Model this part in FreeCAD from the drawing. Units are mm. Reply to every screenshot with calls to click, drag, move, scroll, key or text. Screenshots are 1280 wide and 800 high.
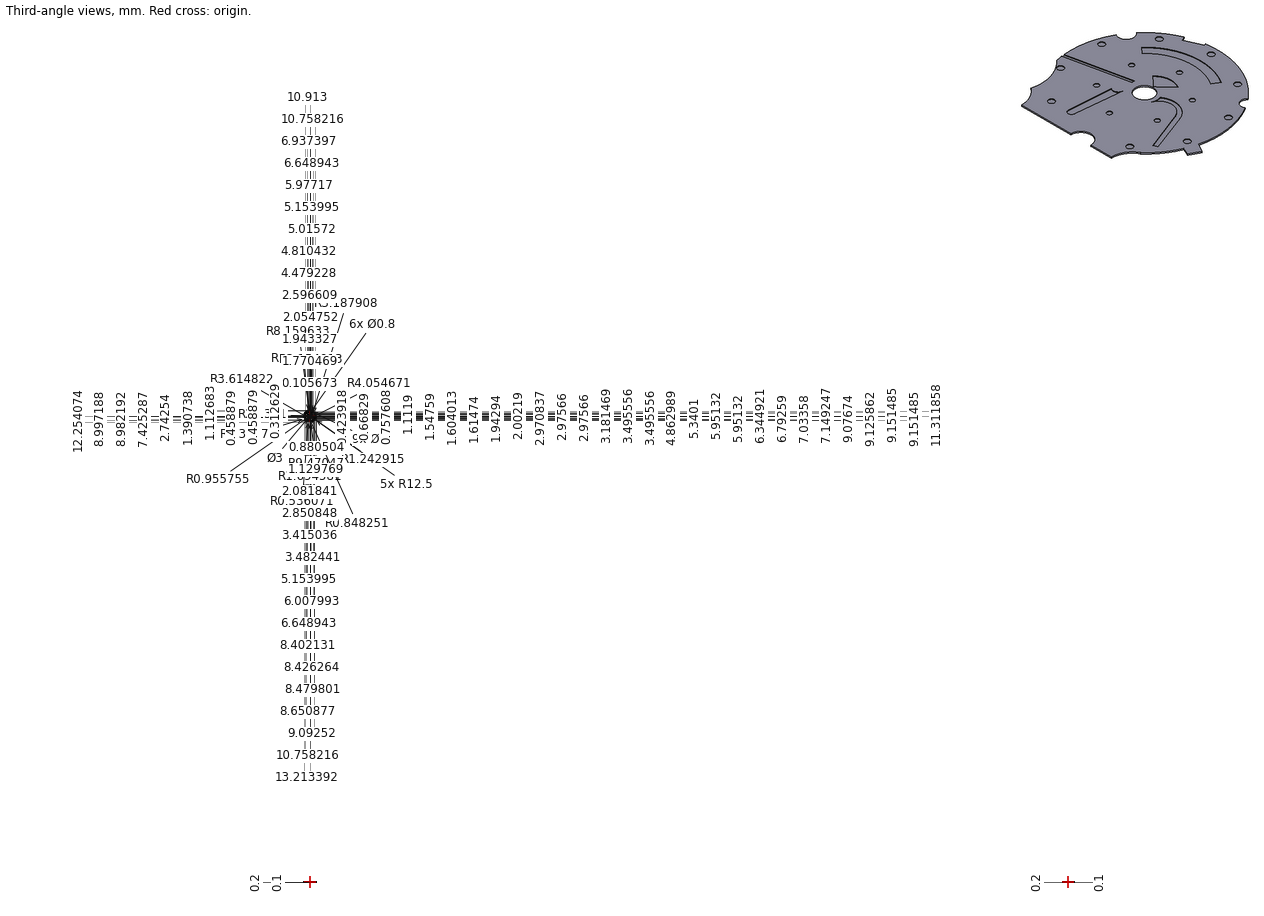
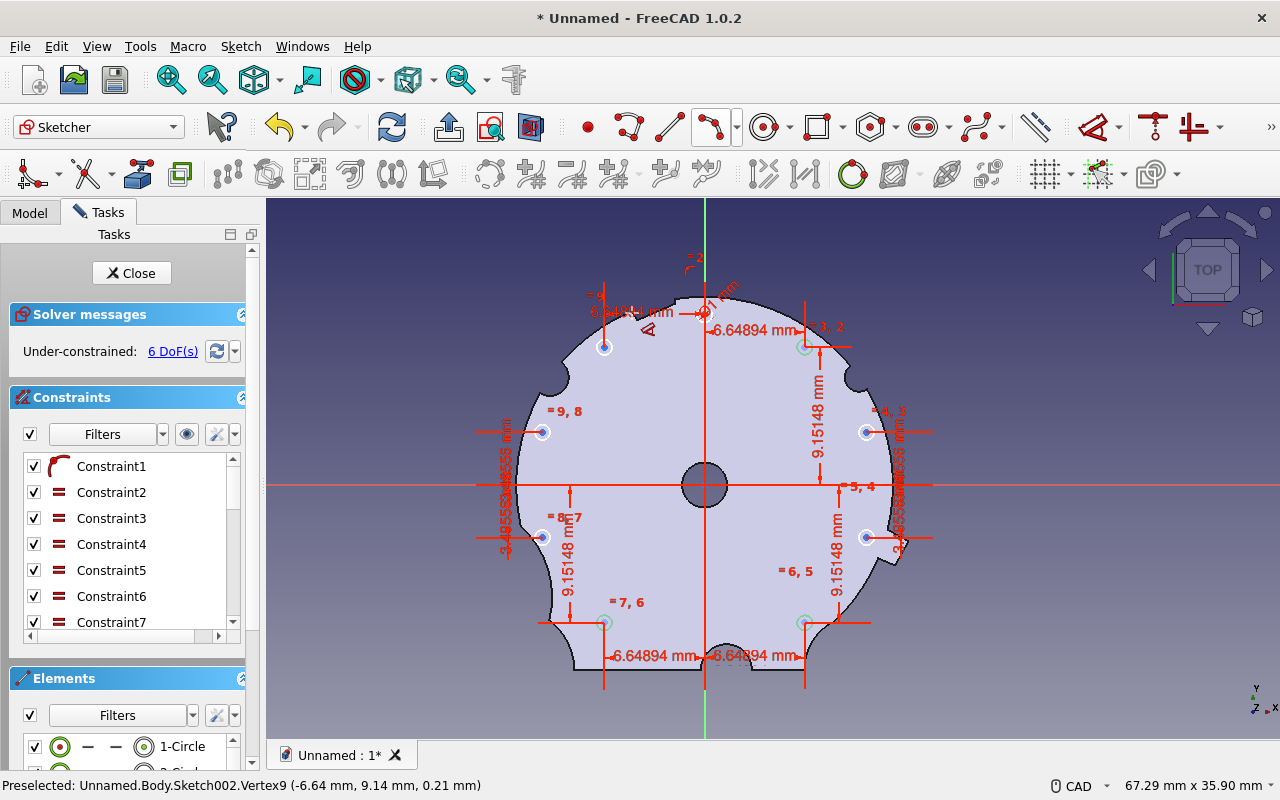
click(604, 347)
click(570, 416)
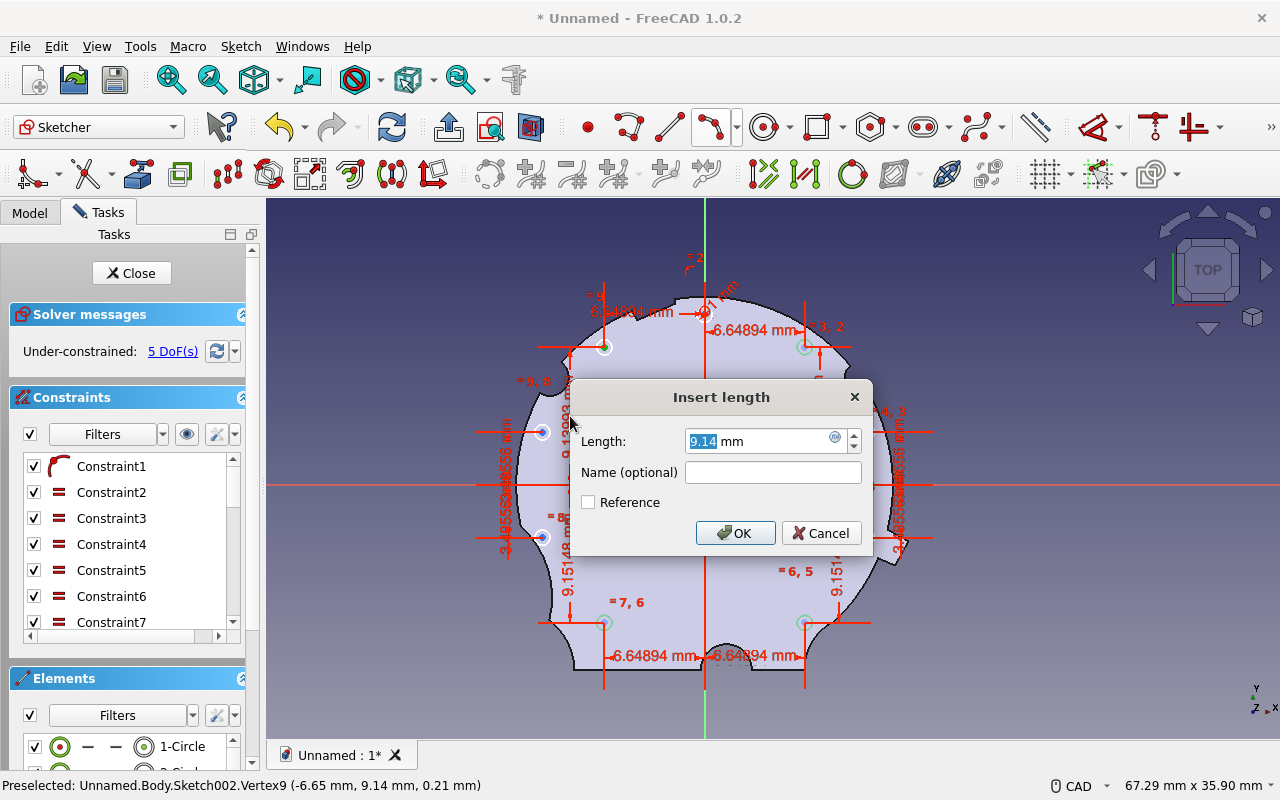
text(9.151485)
key(Return)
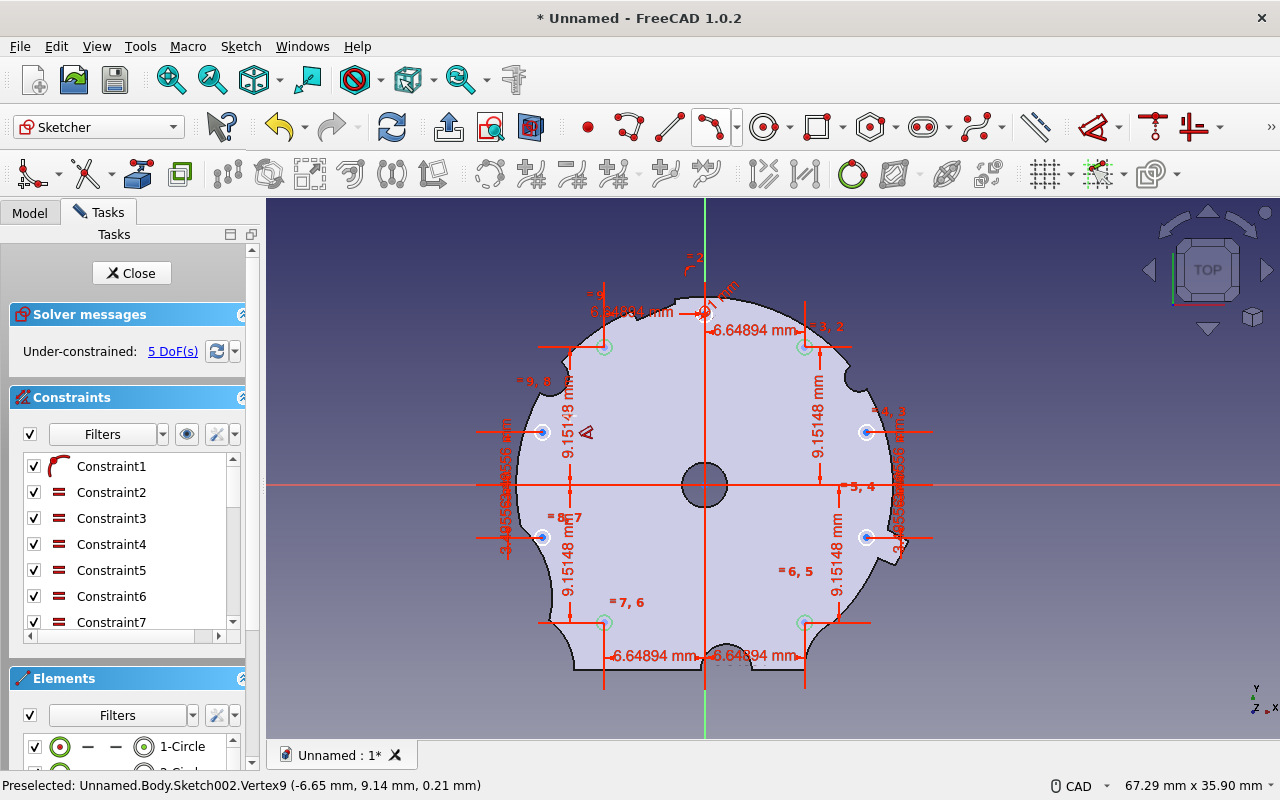
click(705, 315)
click(739, 400)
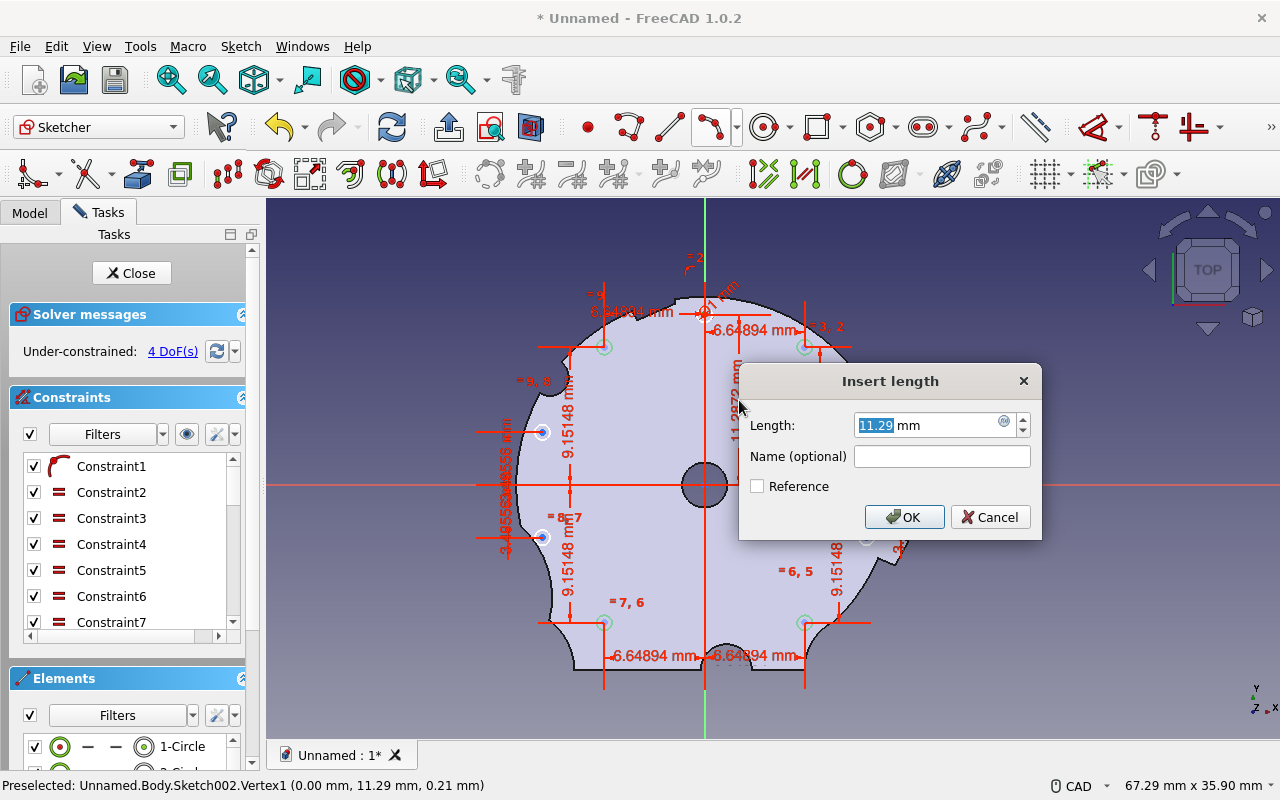
text(11.311858)
key(Return)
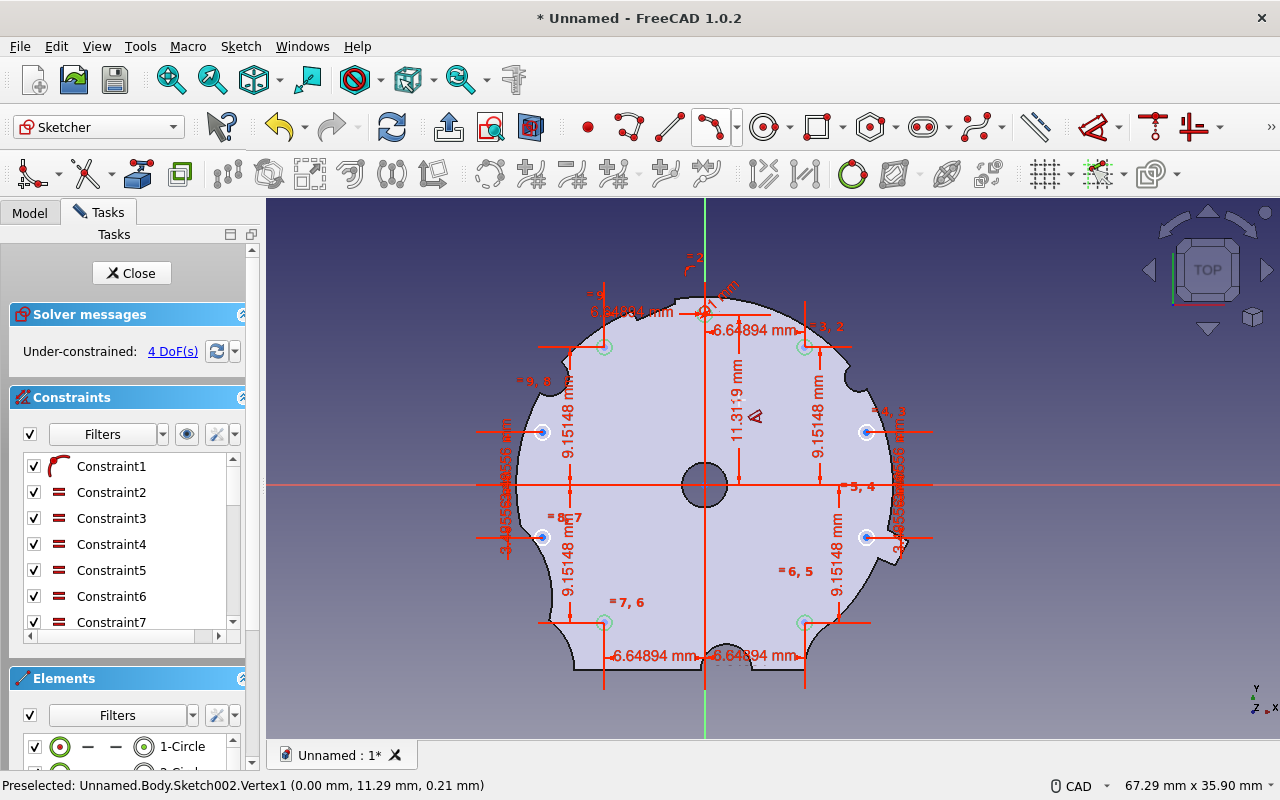
click(867, 432)
click(786, 519)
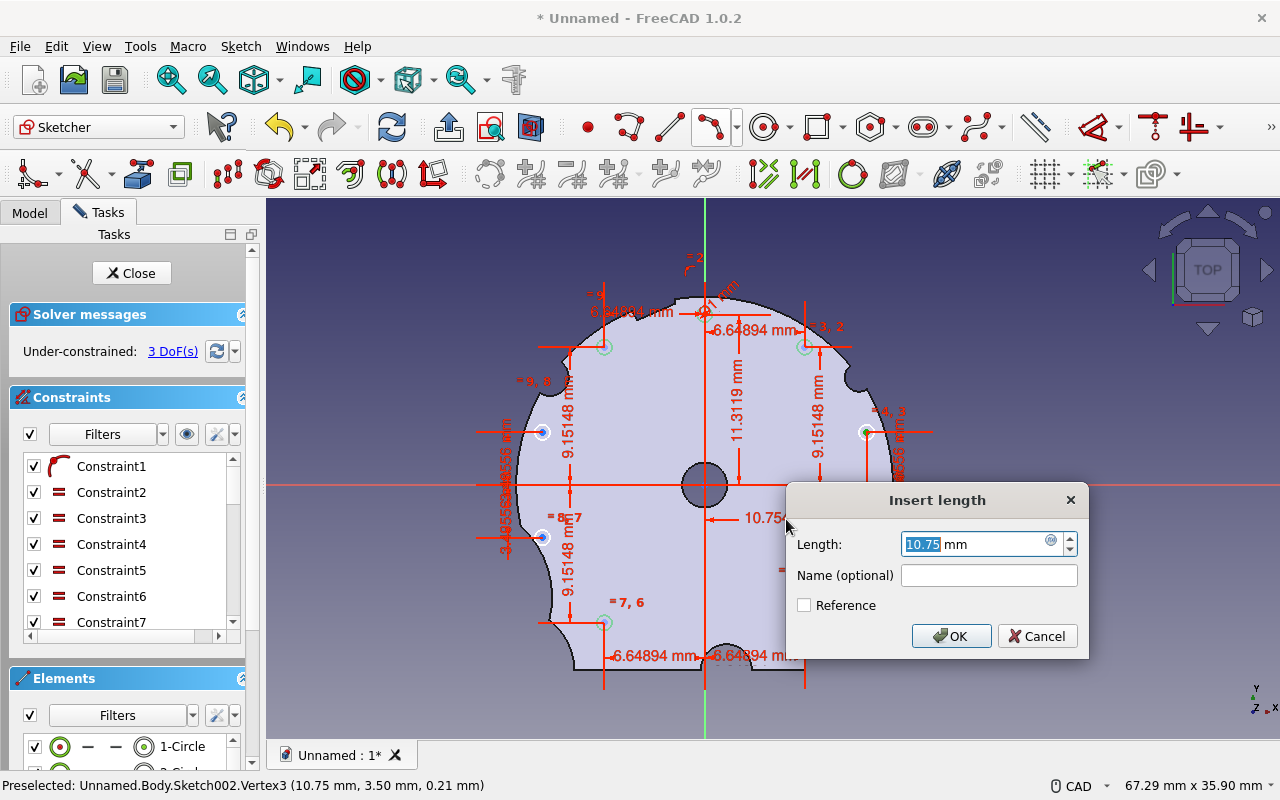
text(10.758216)
key(Return)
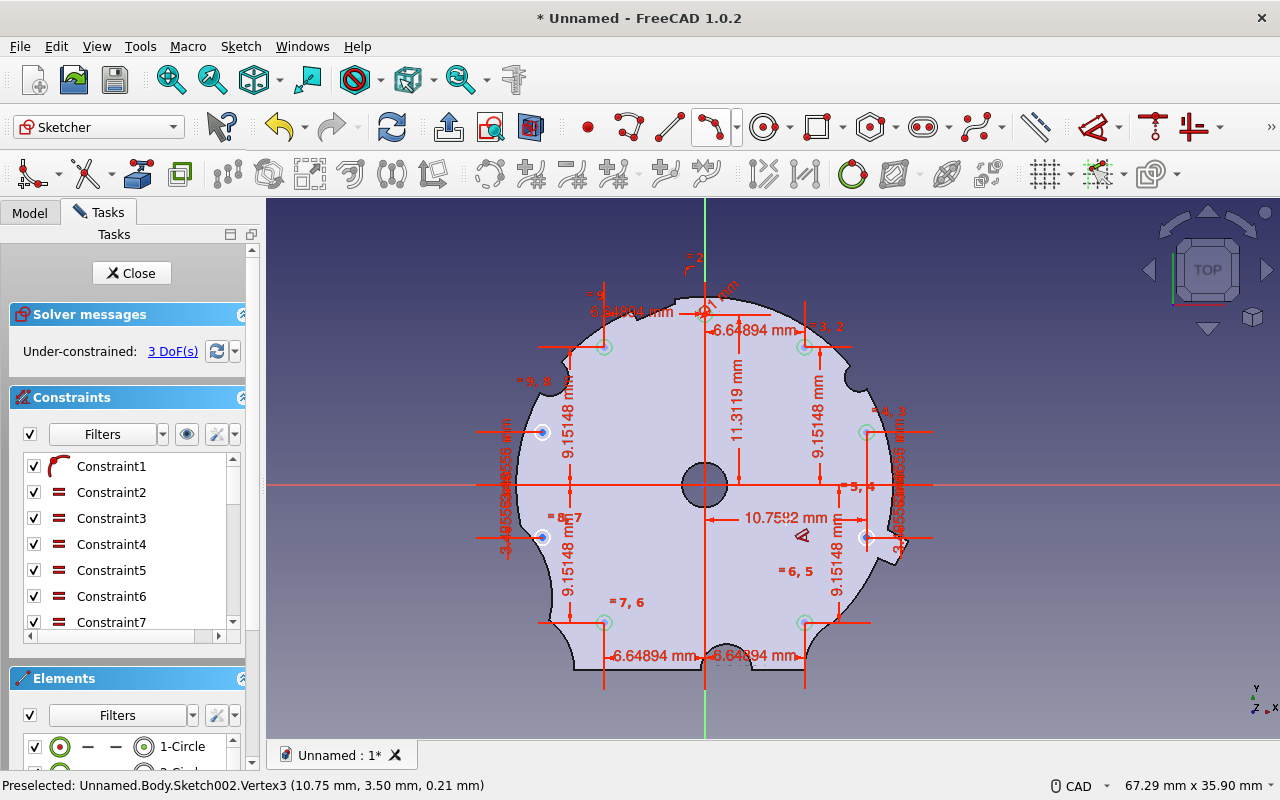
click(867, 538)
click(748, 572)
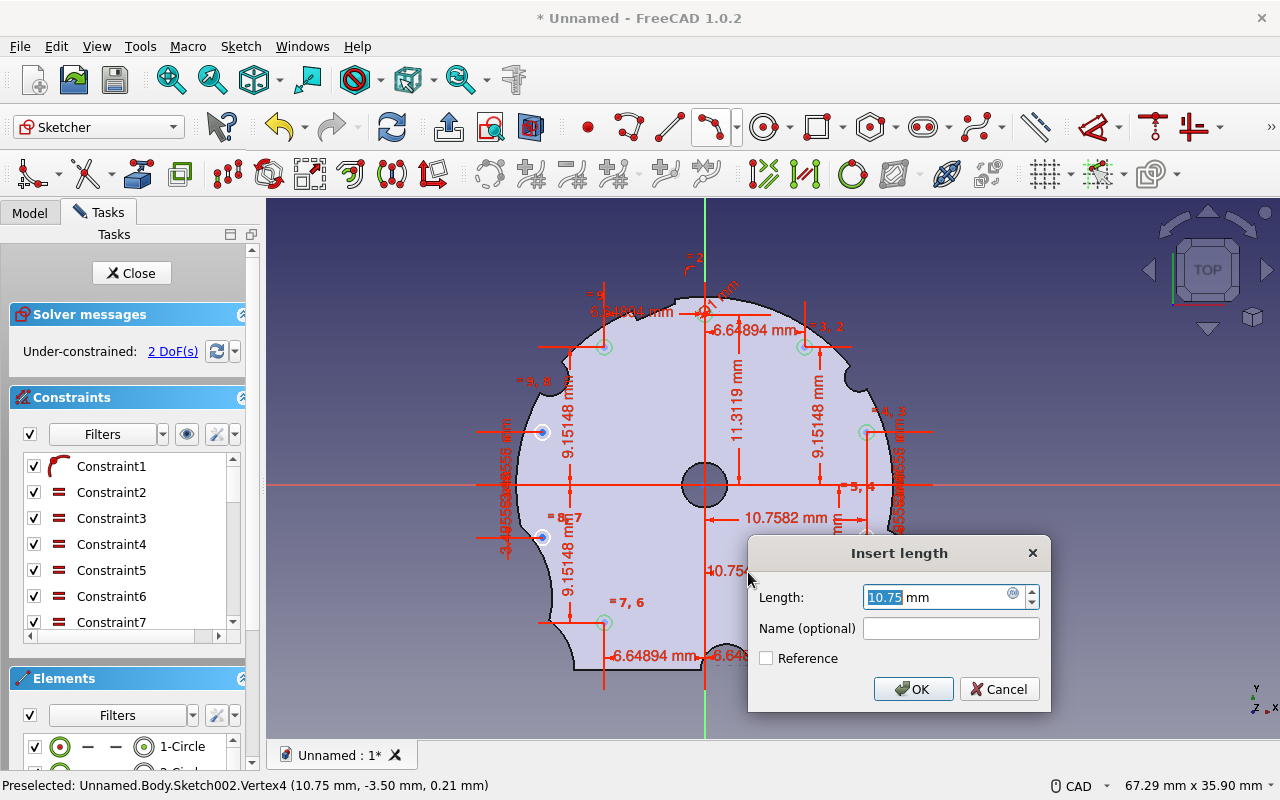
text(10.758216)
key(Return)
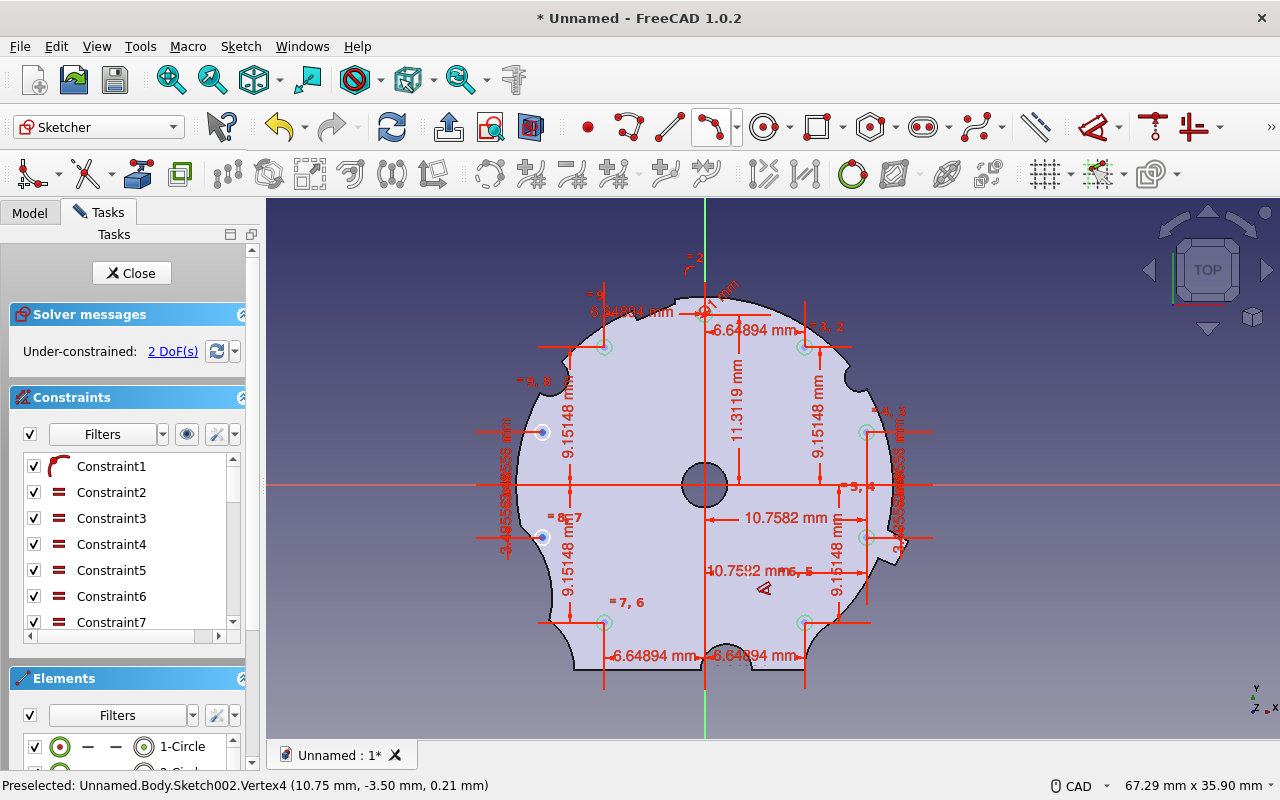
click(542, 538)
click(661, 572)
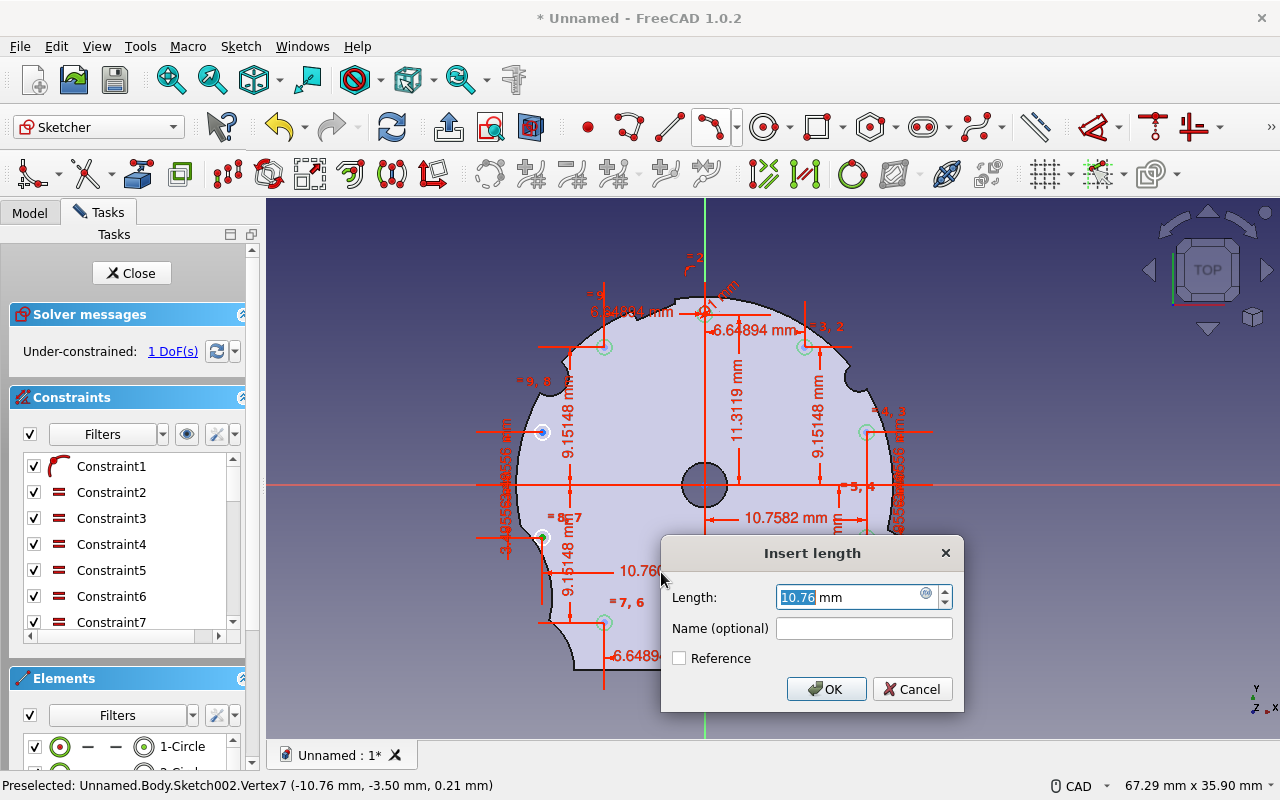
text(10.758216)
key(Return)